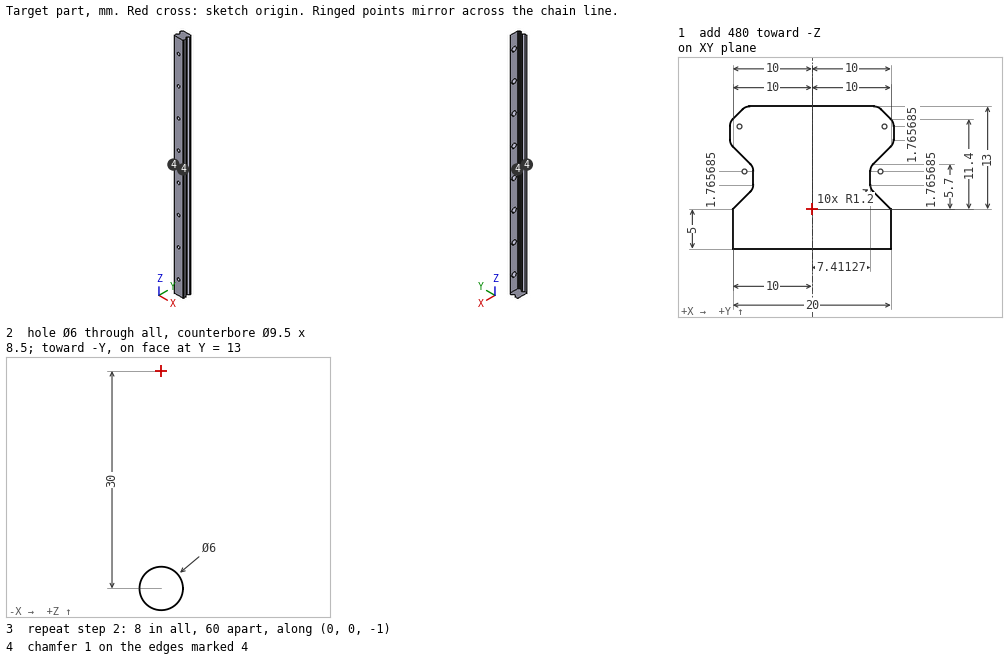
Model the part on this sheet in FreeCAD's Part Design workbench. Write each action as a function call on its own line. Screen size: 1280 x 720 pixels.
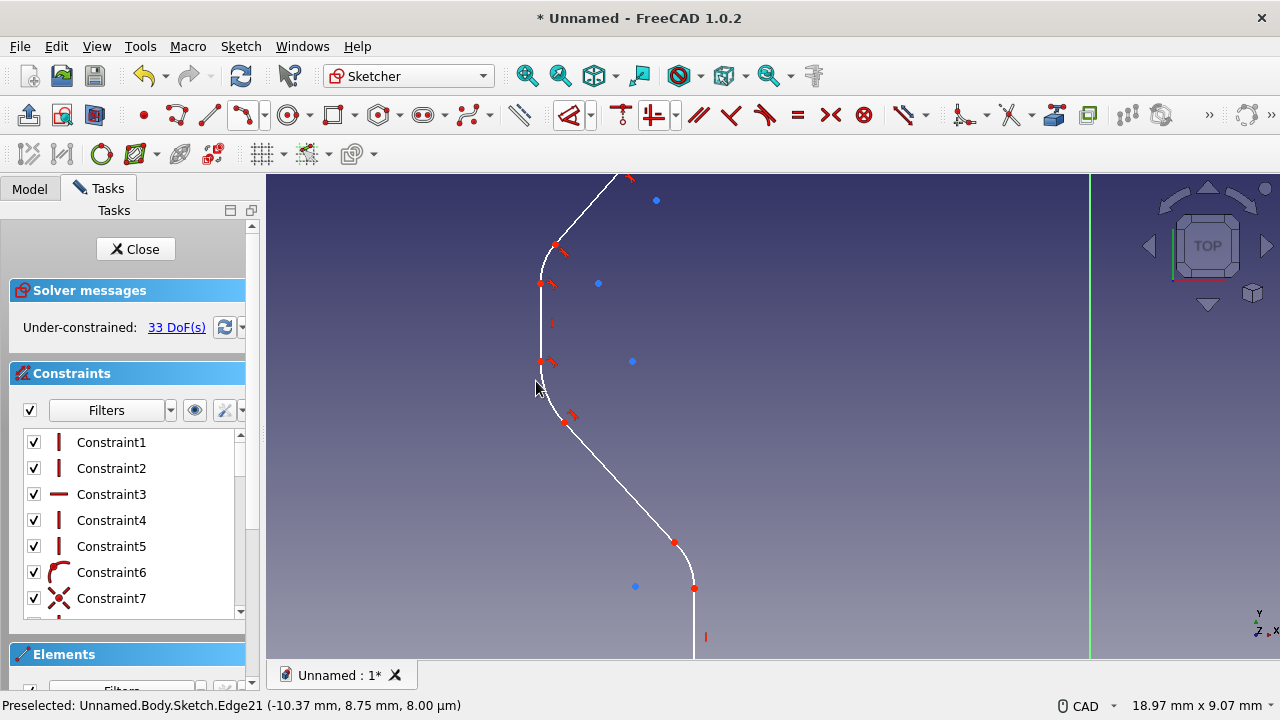
click(597, 459)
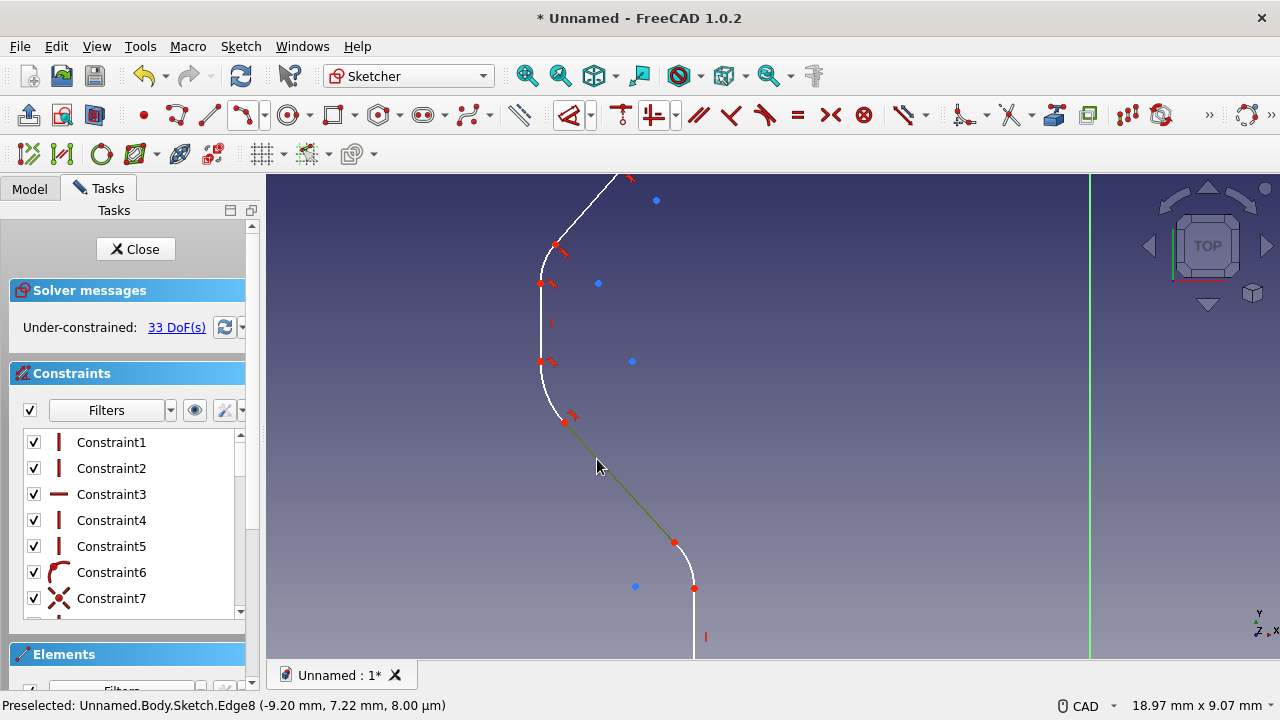
click(692, 573)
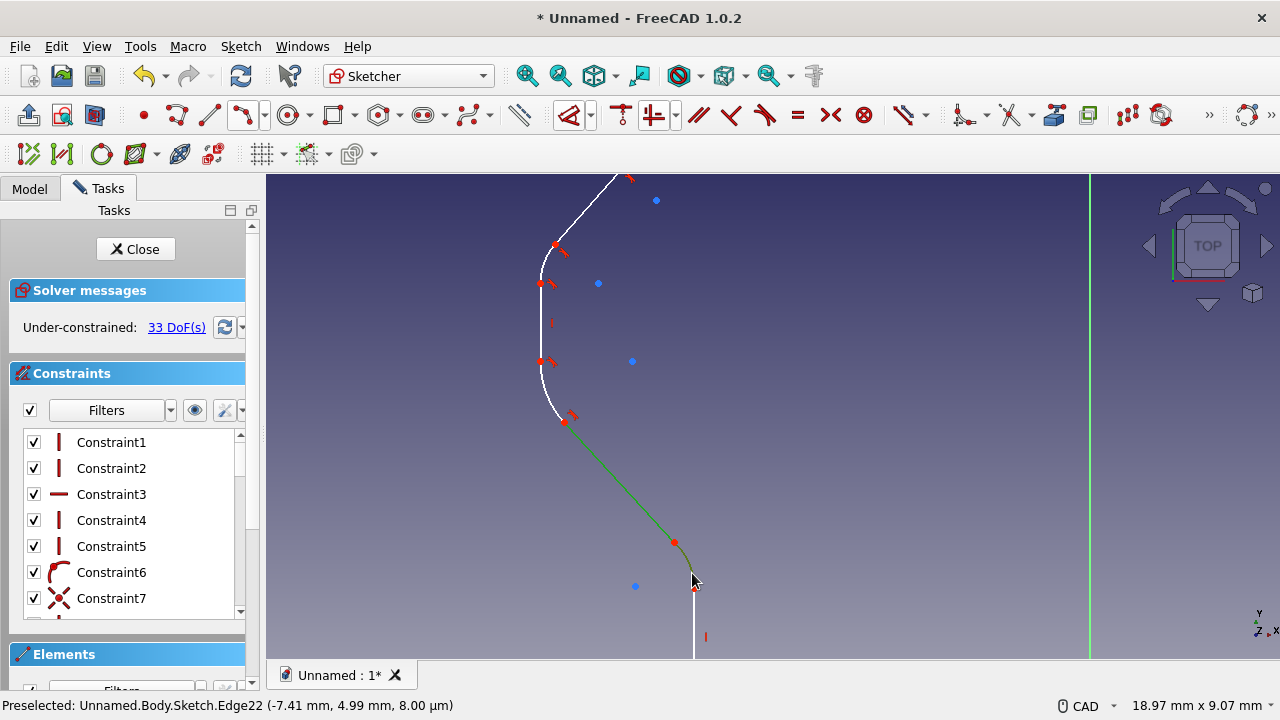
key(t)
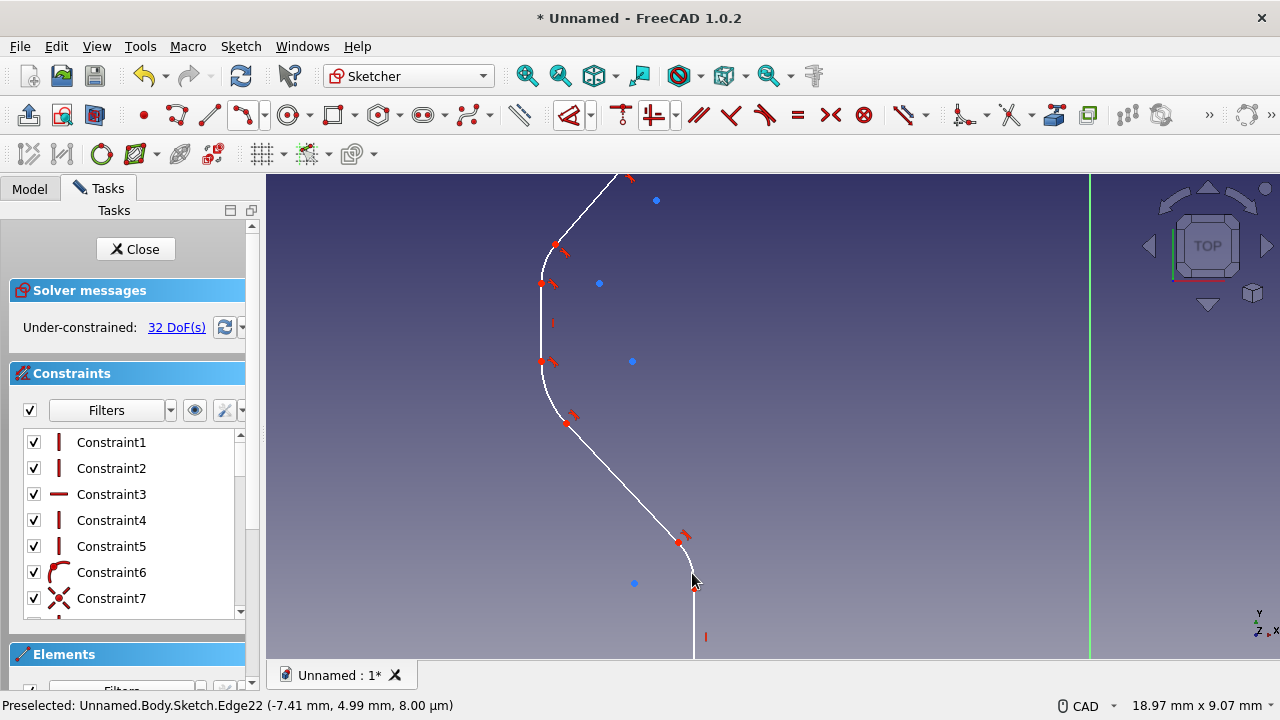
click(694, 617)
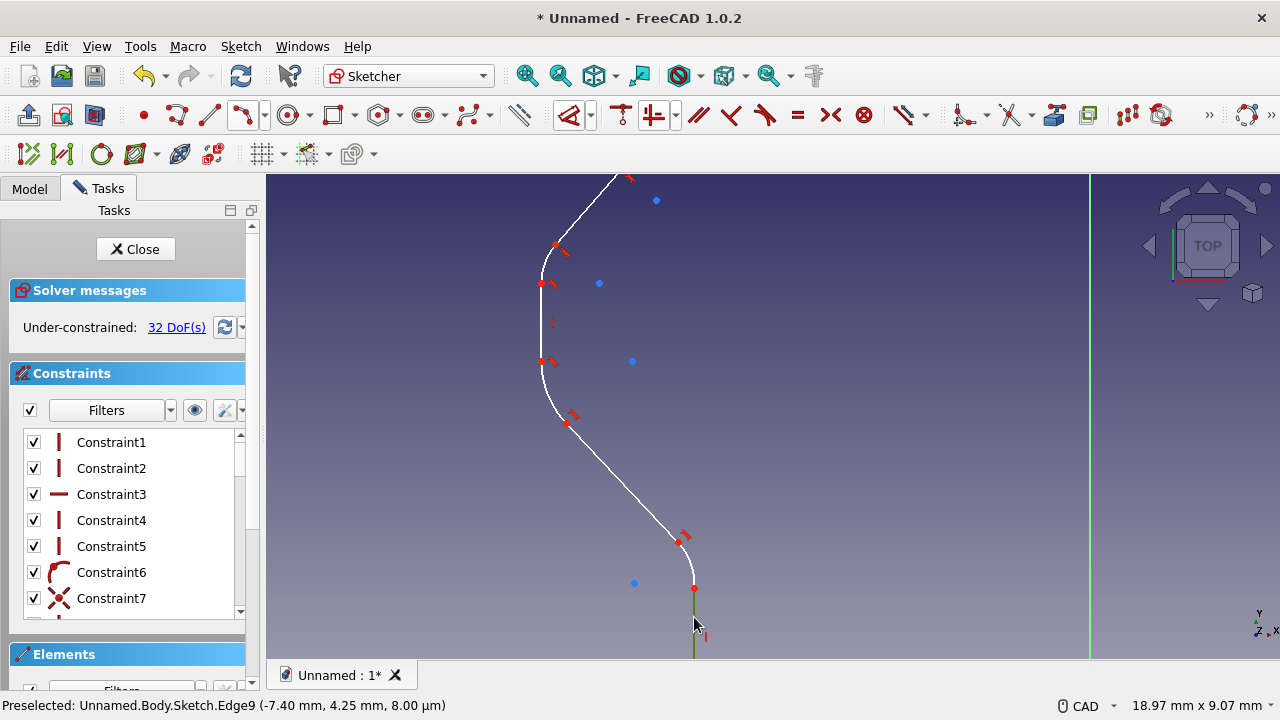
click(693, 574)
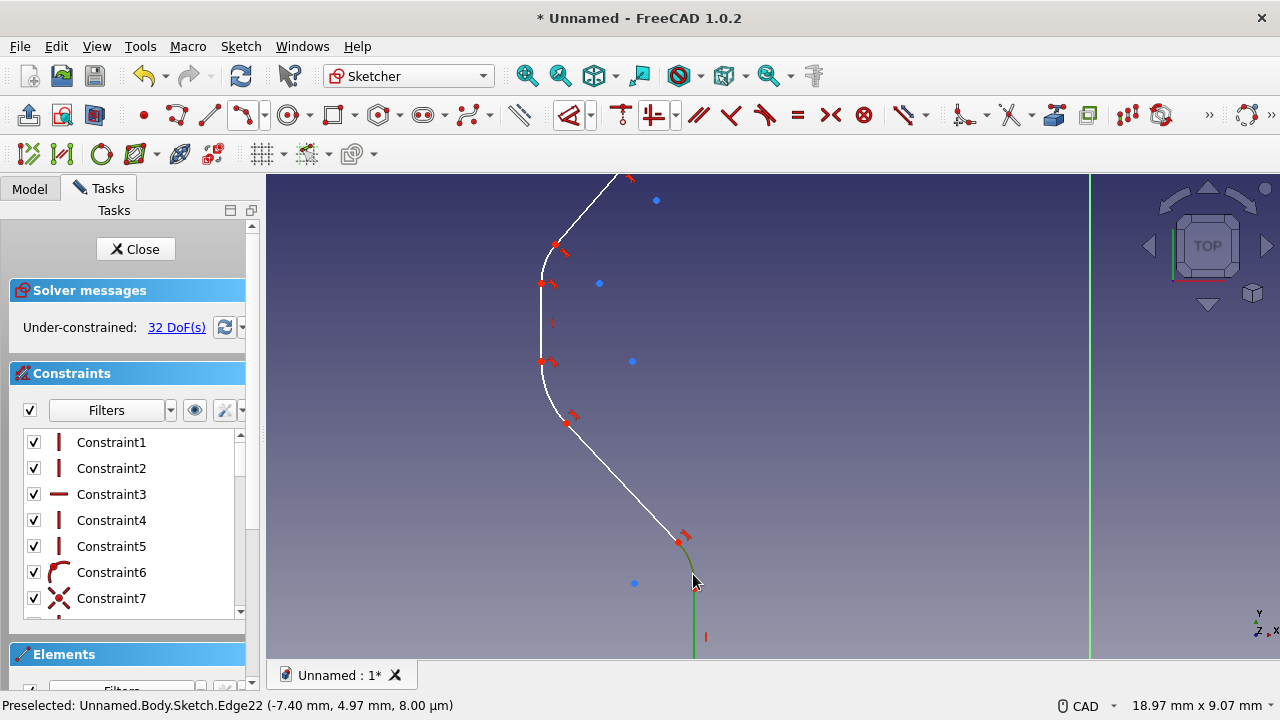
key(t)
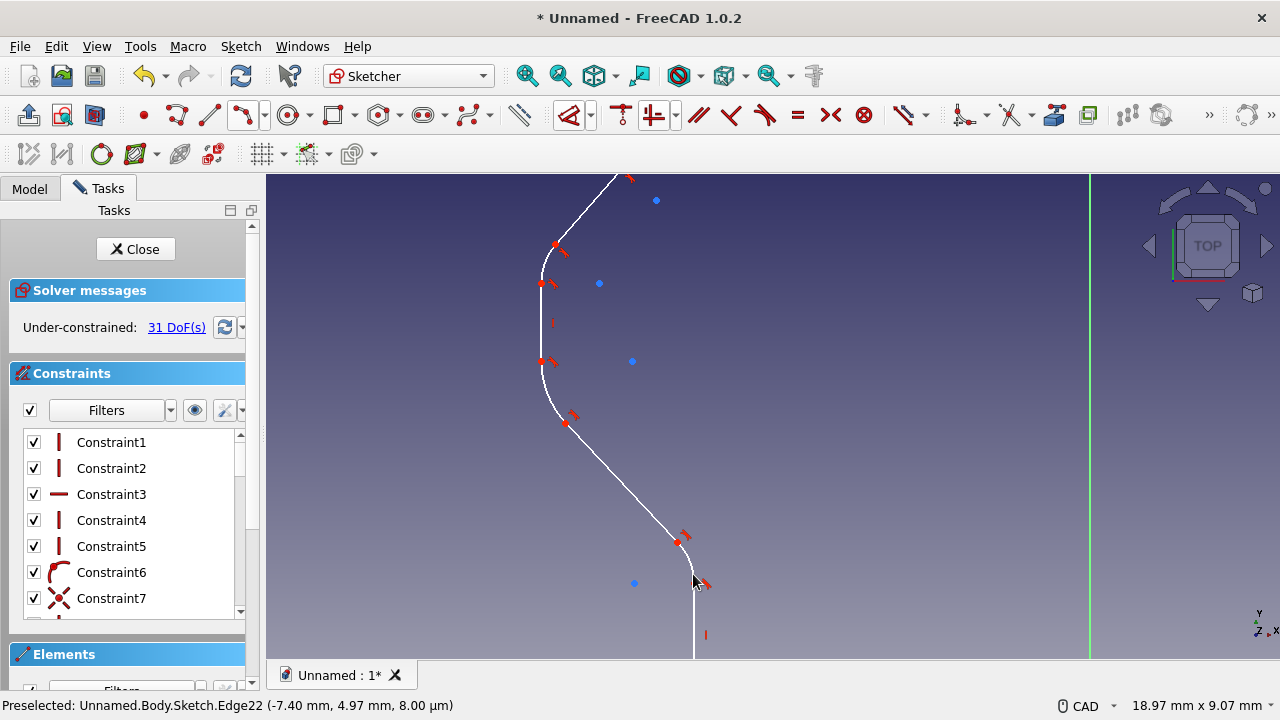
click(694, 614)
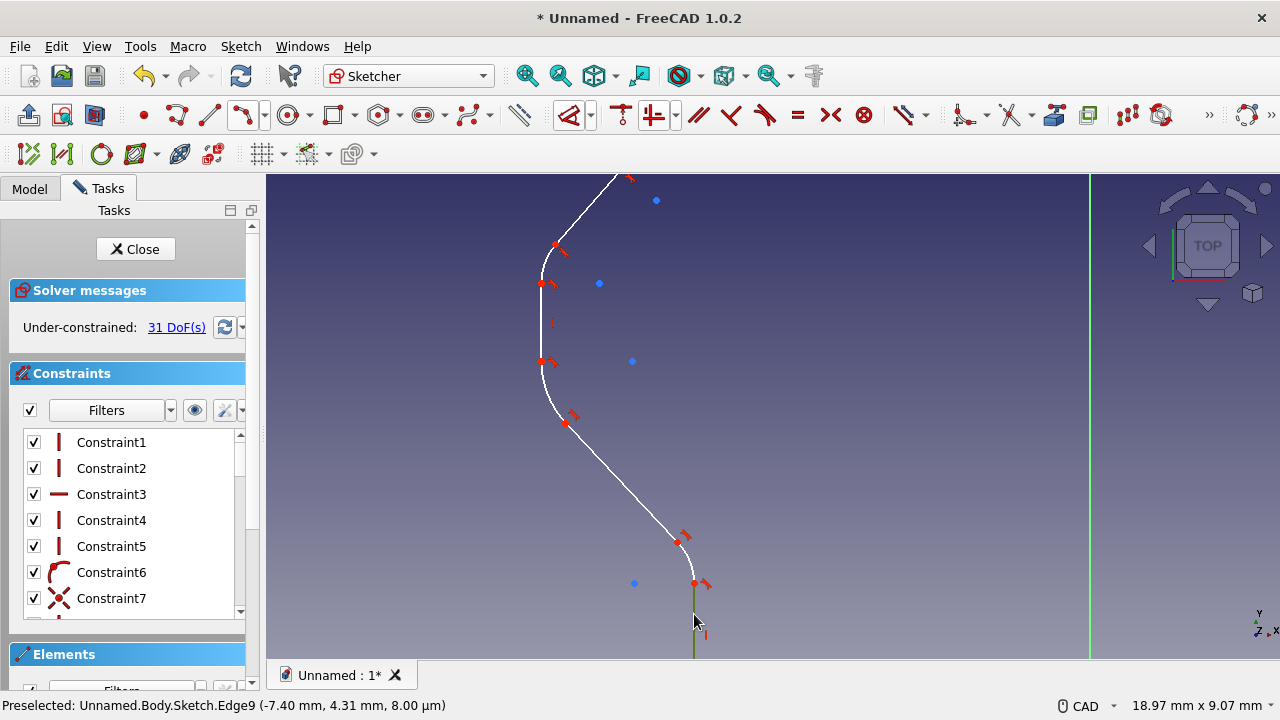
scroll(538, 324, down, 6)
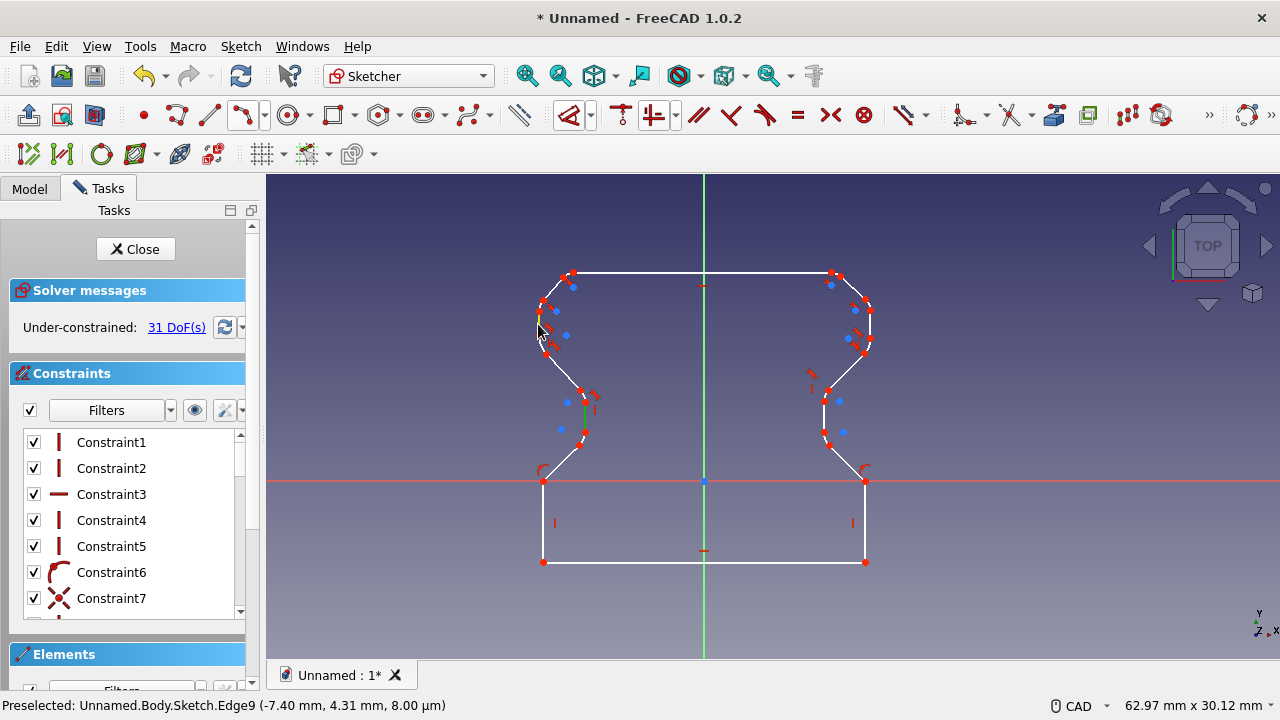
scroll(582, 442, up, 6)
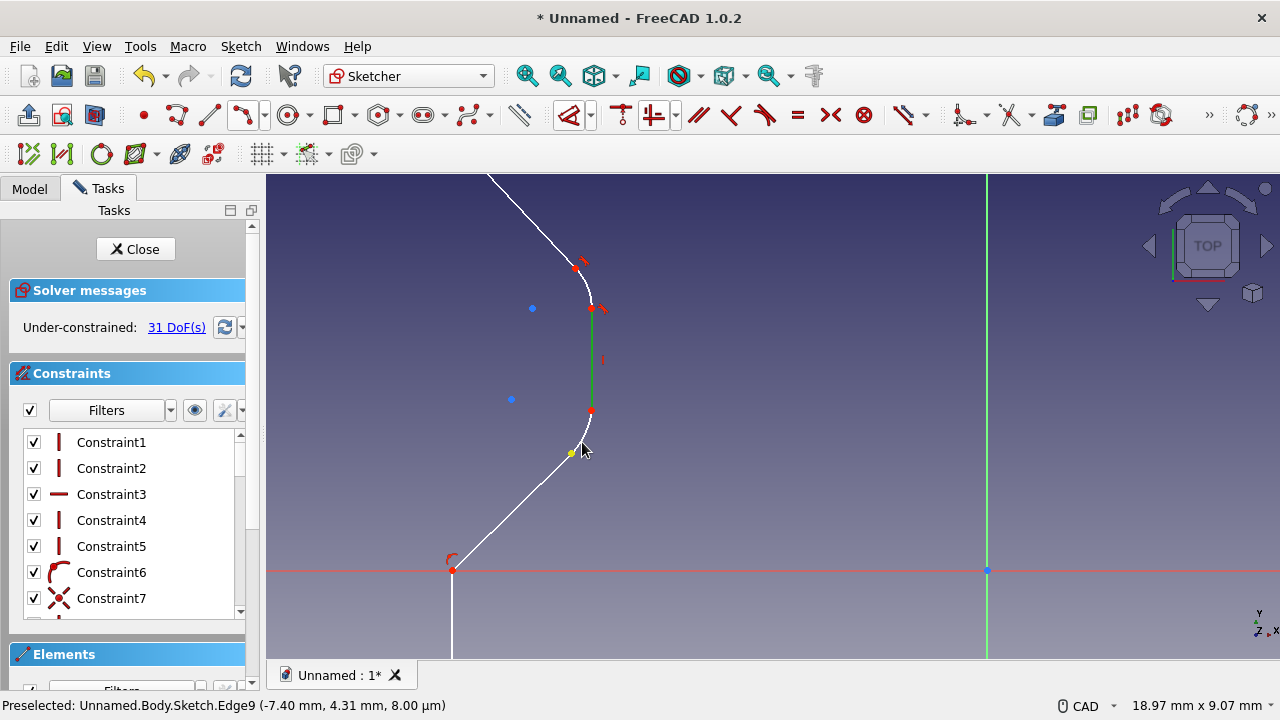
click(581, 442)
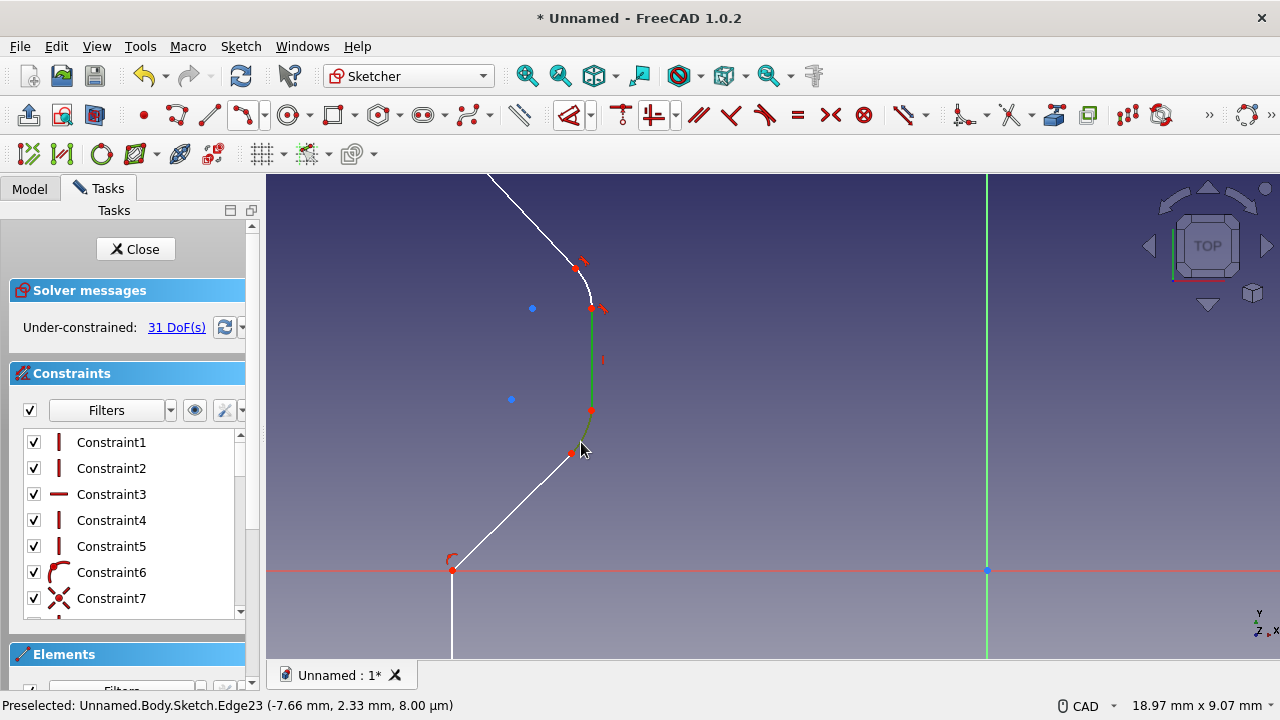
key(t)